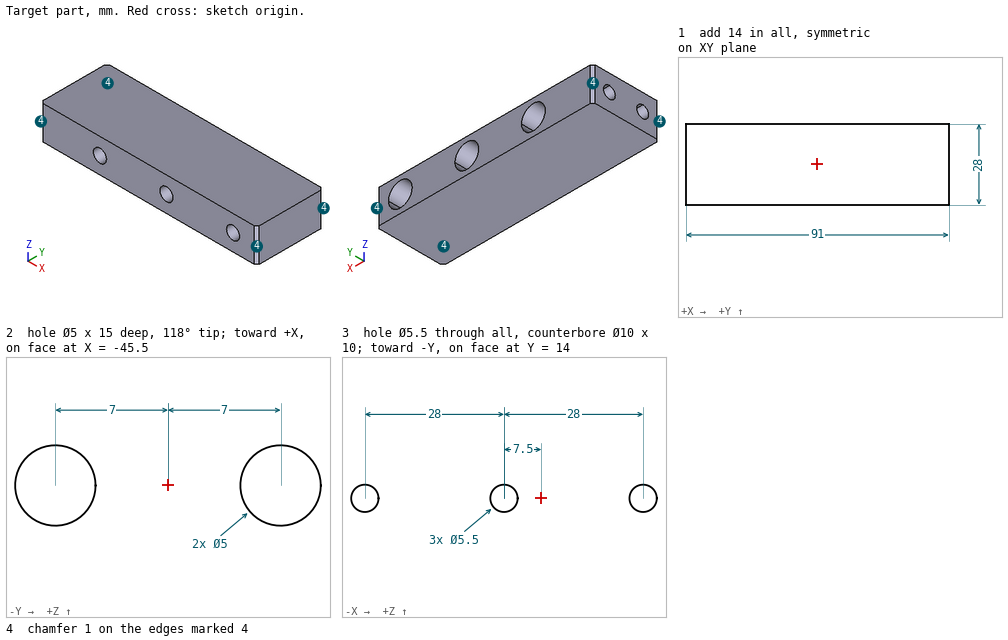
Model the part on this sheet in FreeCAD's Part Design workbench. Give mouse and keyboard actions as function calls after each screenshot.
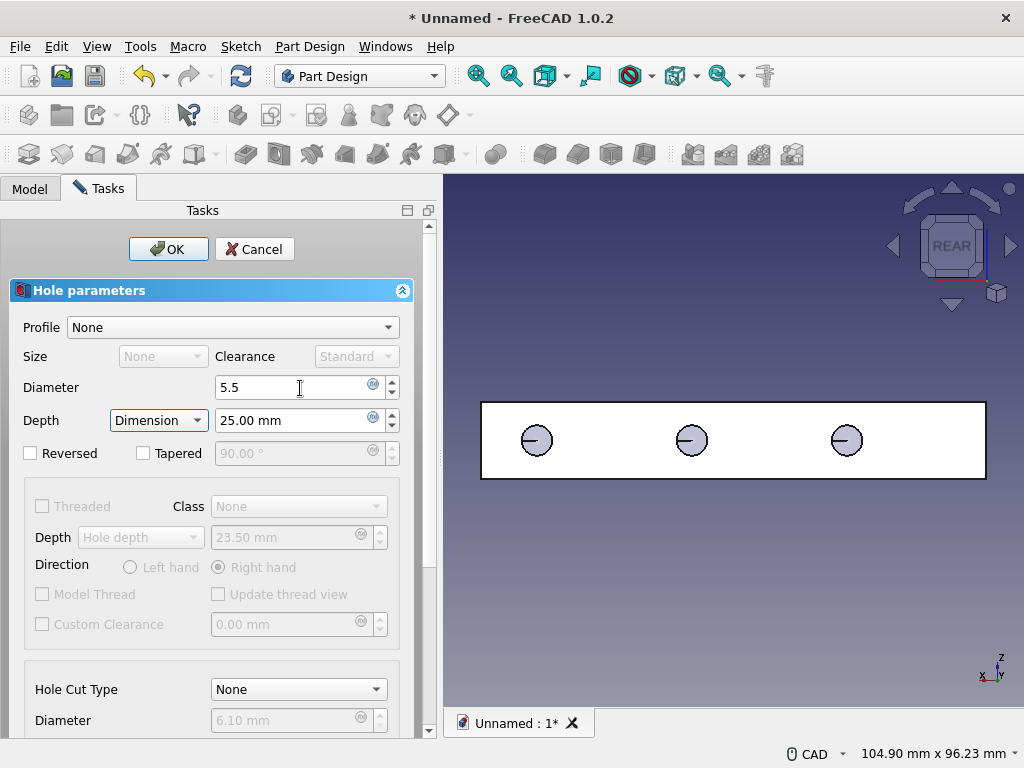
click(160, 420)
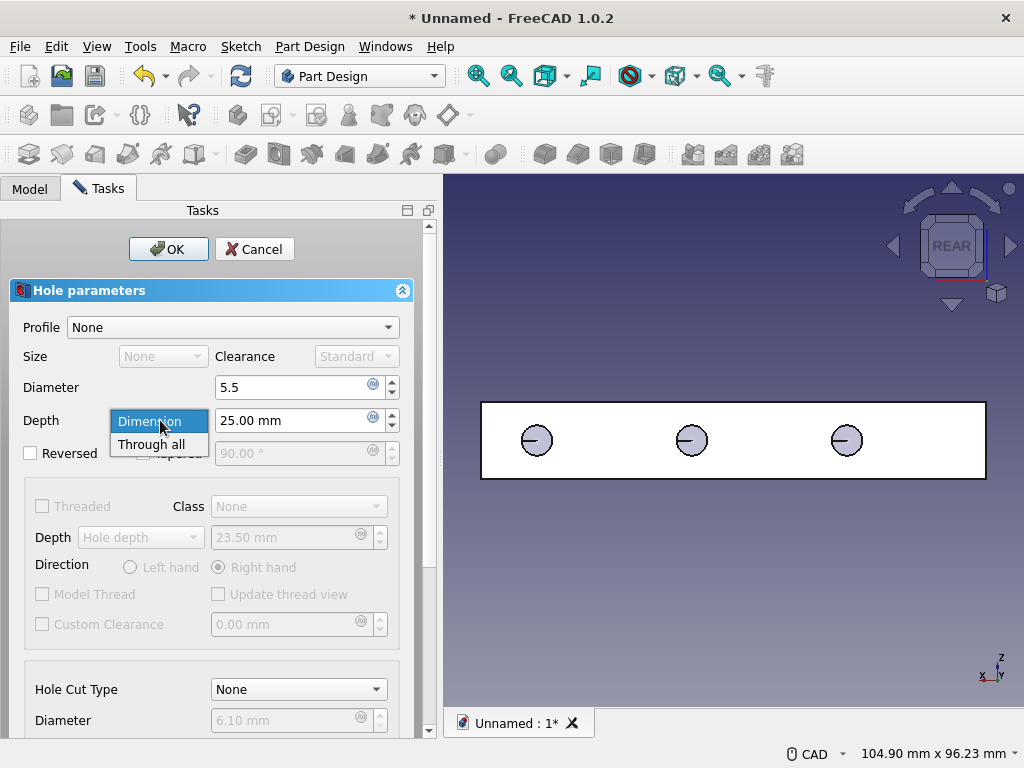
click(158, 444)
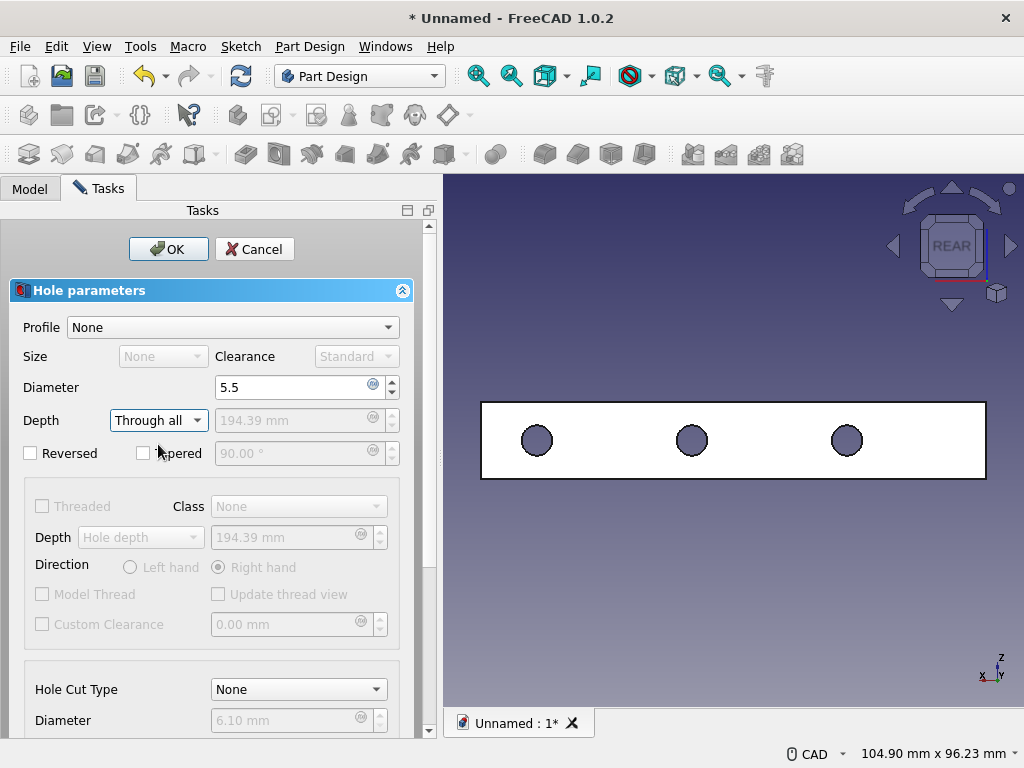
click(300, 690)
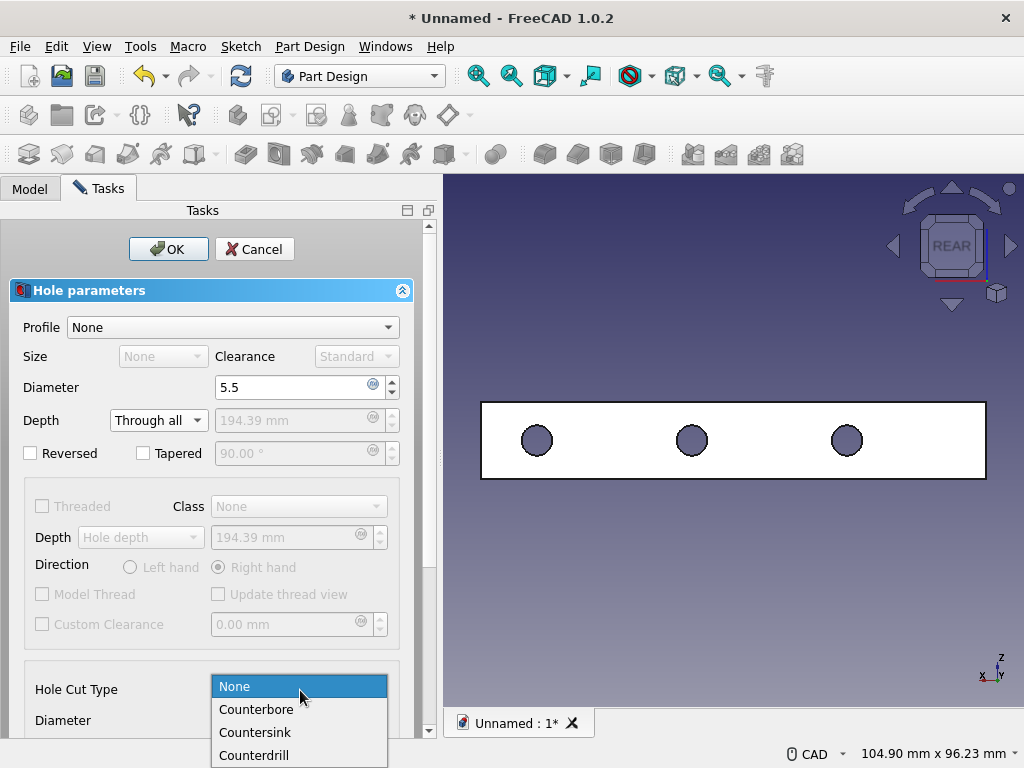
click(298, 710)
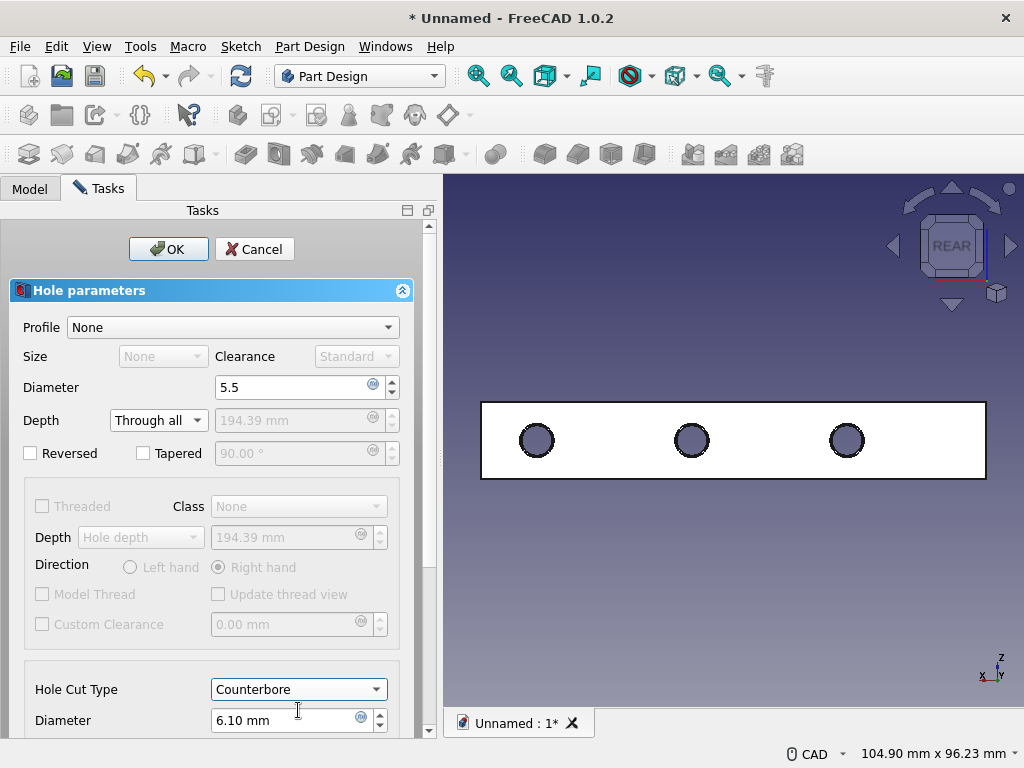
triple_click(292, 720)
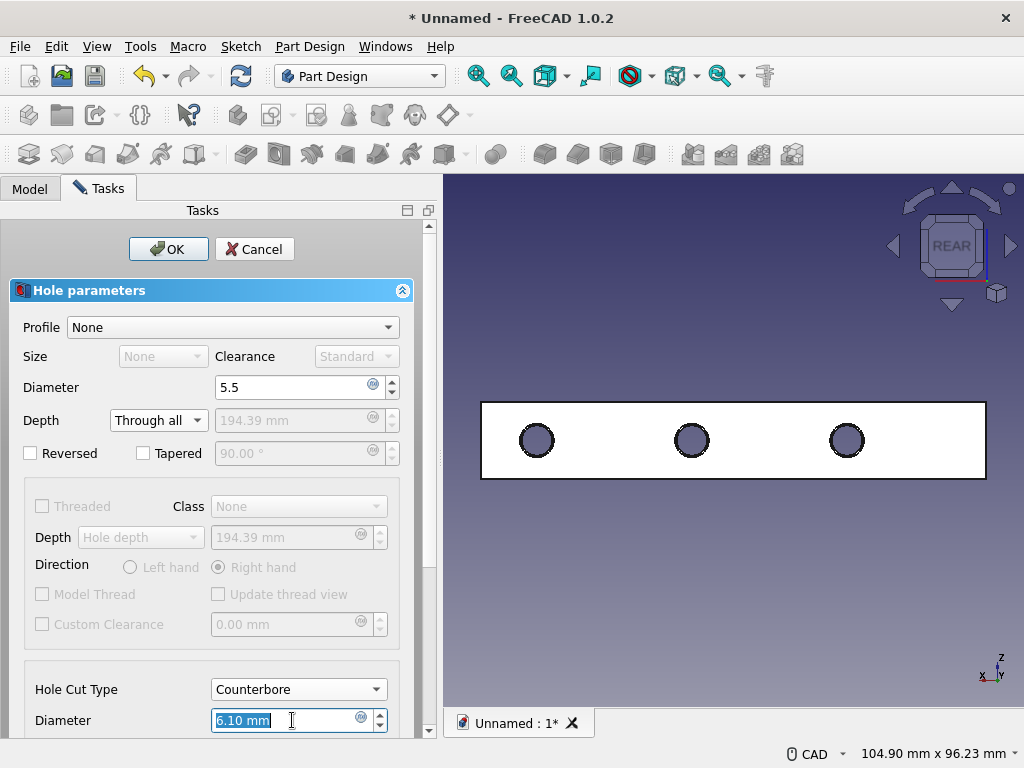
text(10)
key(Tab)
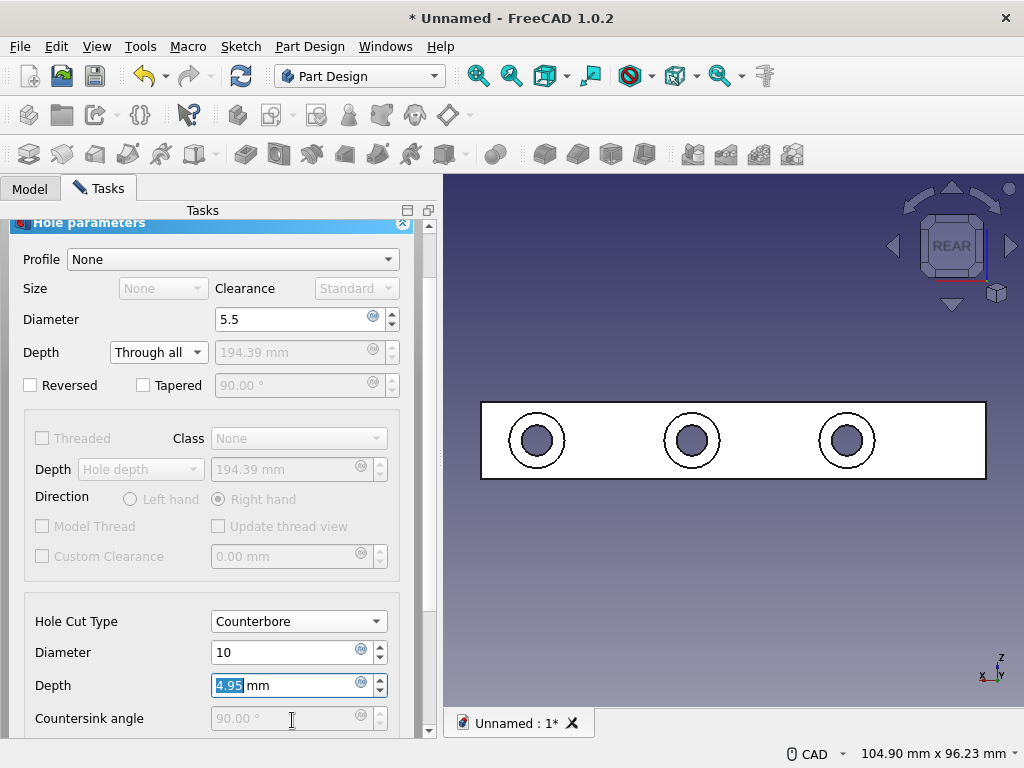
text(10)
key(Tab)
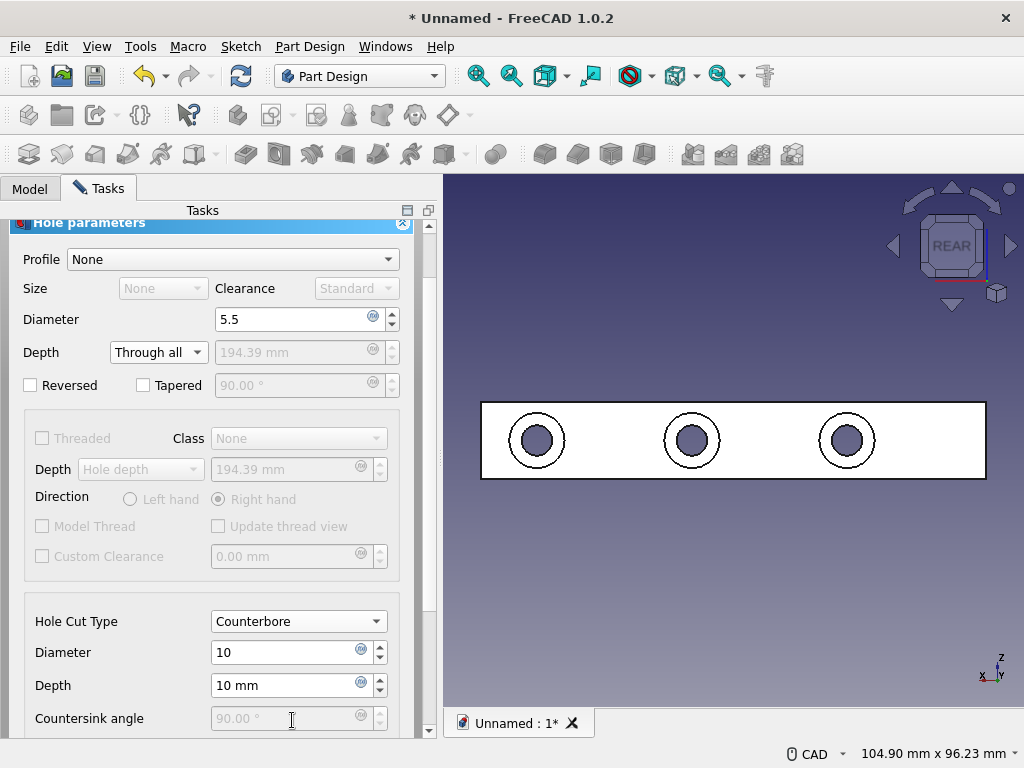
scroll(429, 479, up, 2)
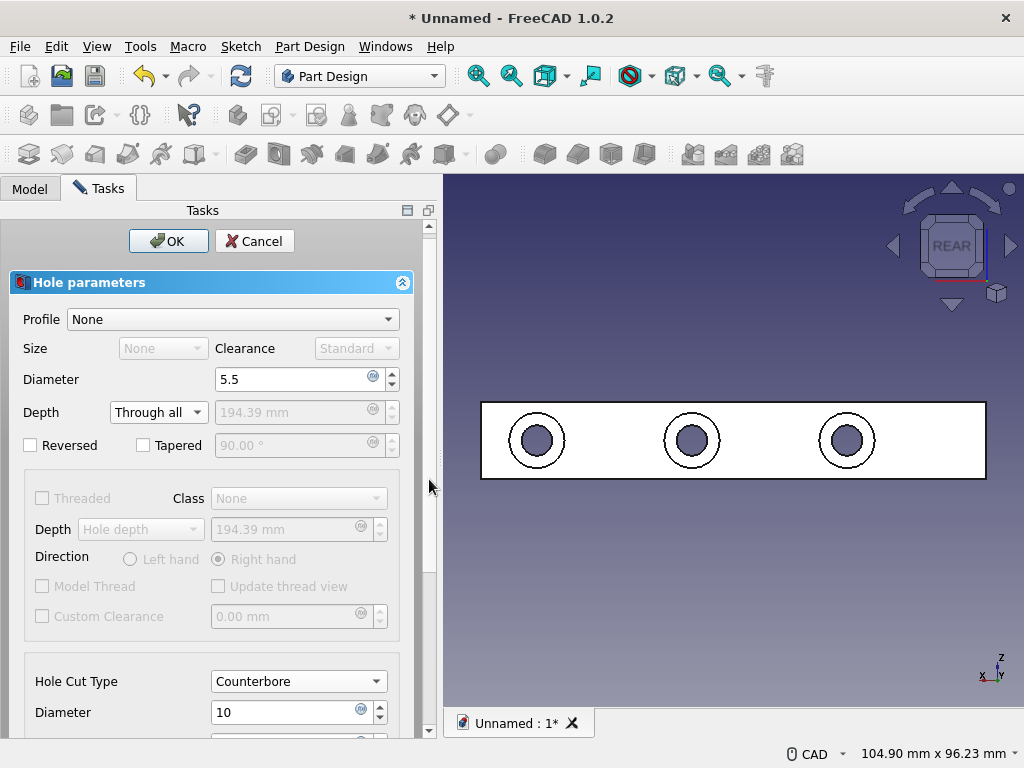
click(169, 249)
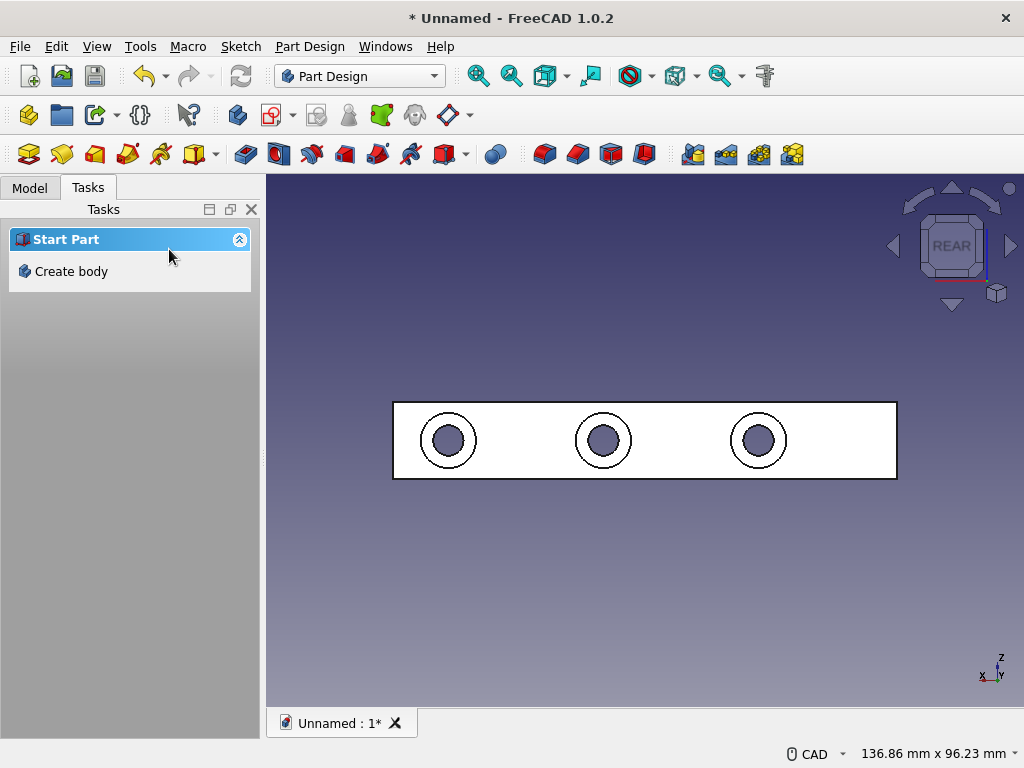
click(897, 440)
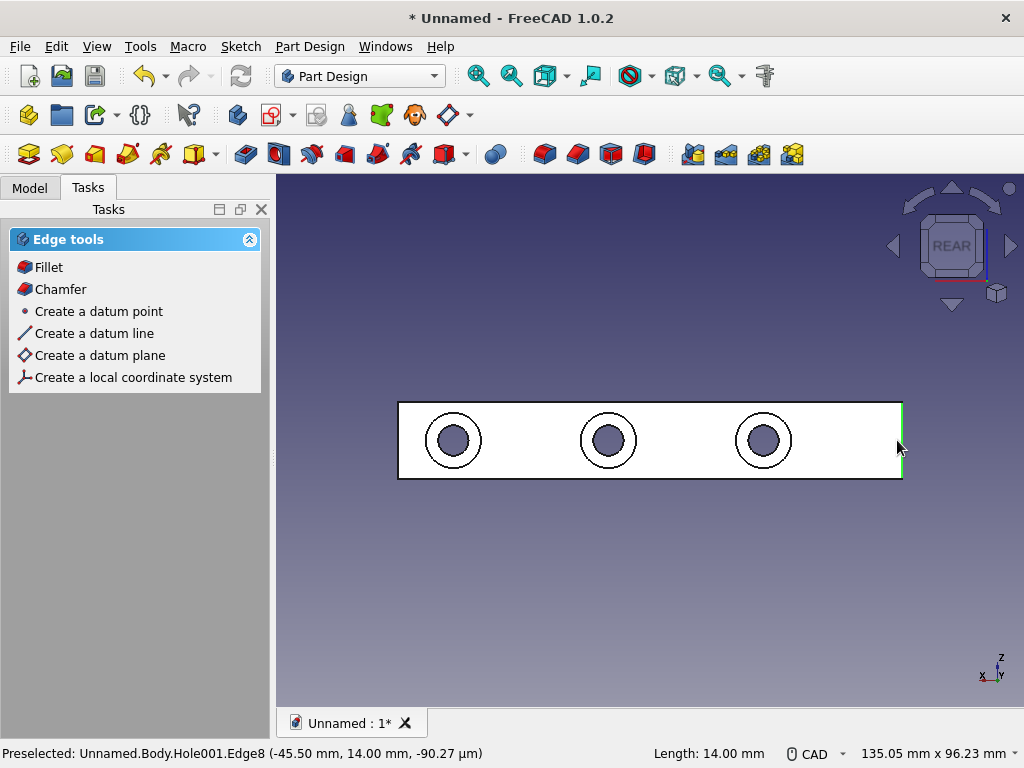
key(0)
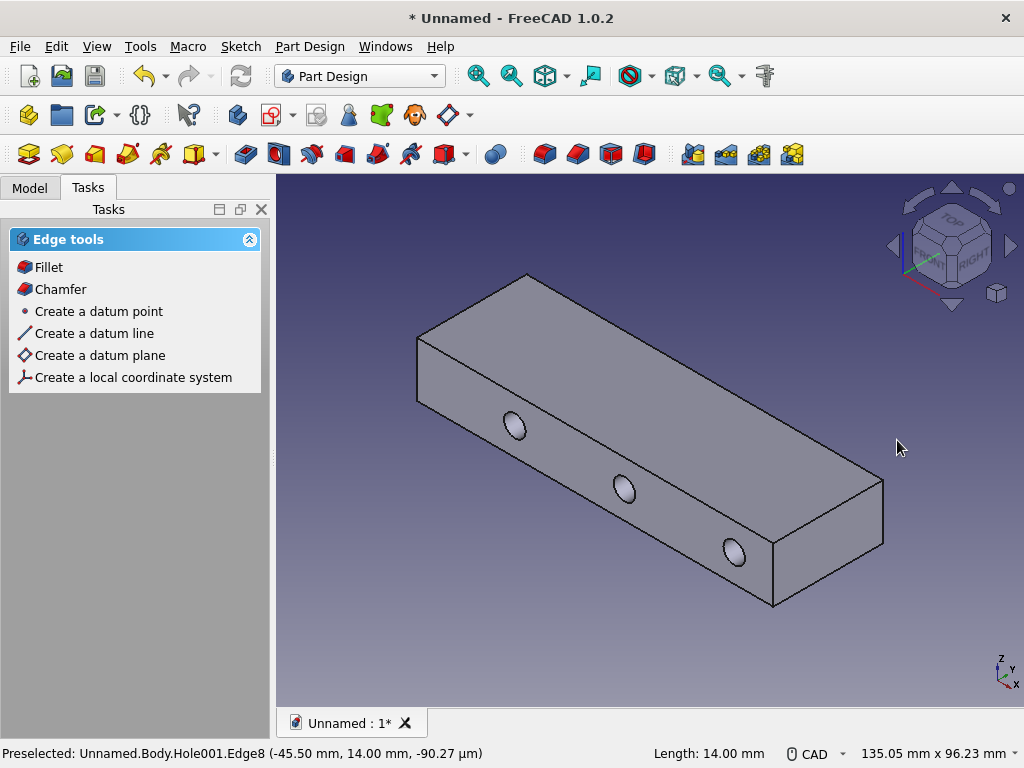
click(773, 574, ctrl)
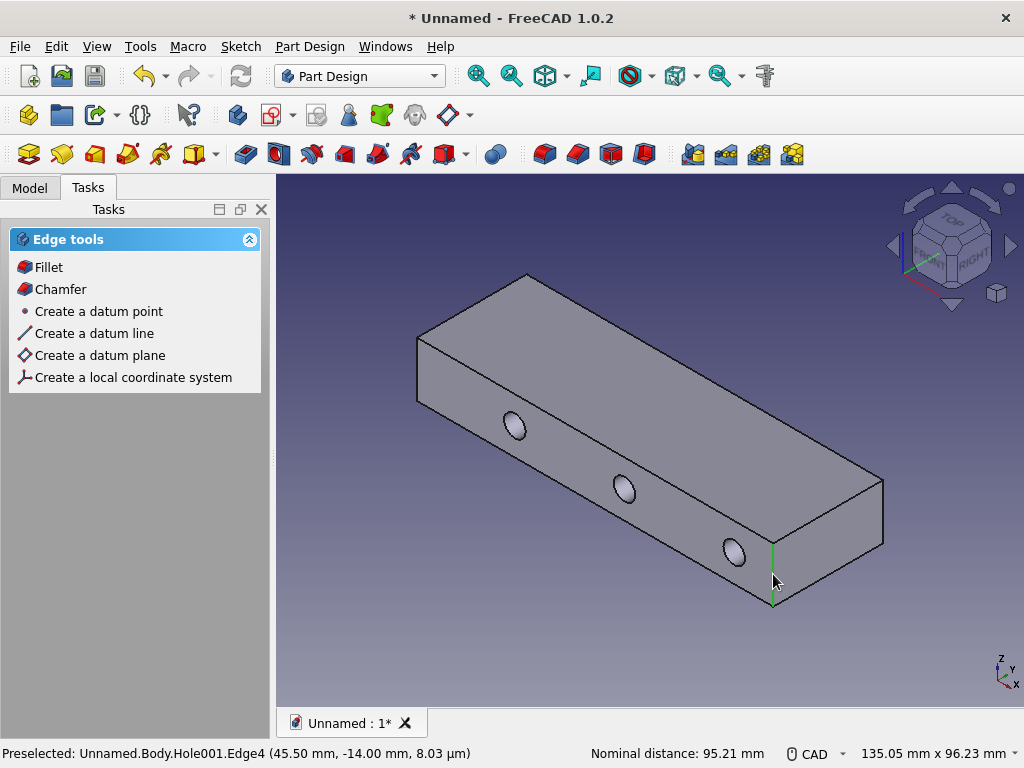
key(2)